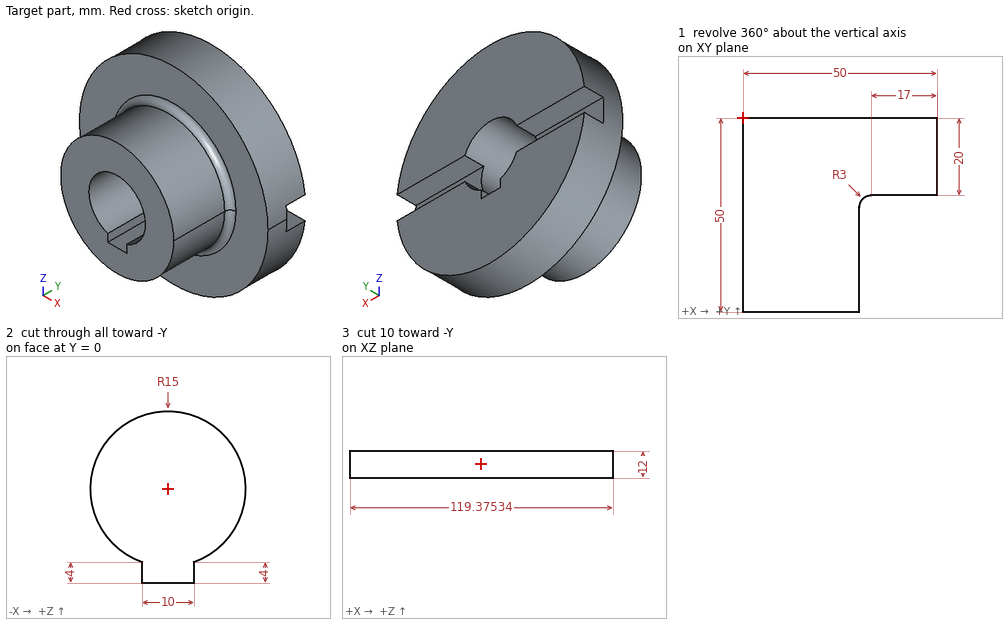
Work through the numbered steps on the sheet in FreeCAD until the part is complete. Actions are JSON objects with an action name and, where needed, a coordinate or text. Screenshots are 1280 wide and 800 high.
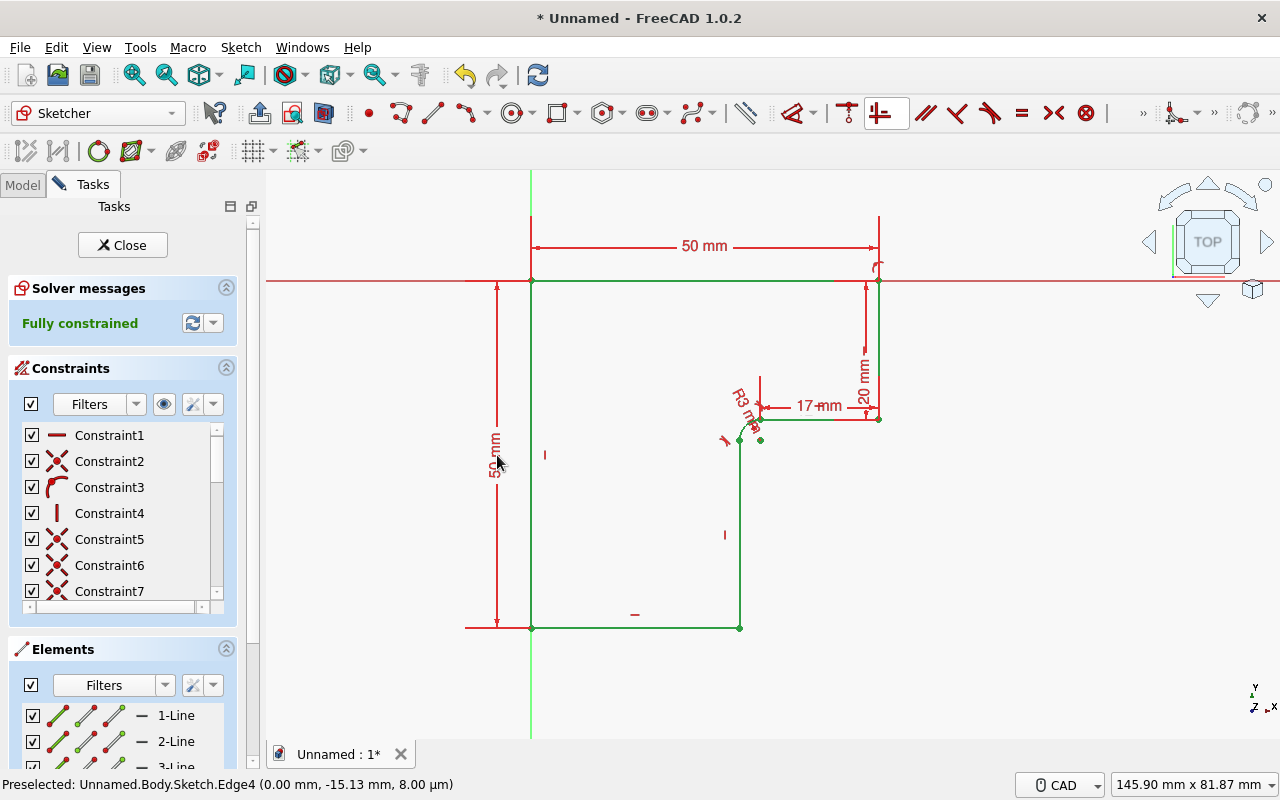
{"action": "left_click", "coordinate": [123, 245]}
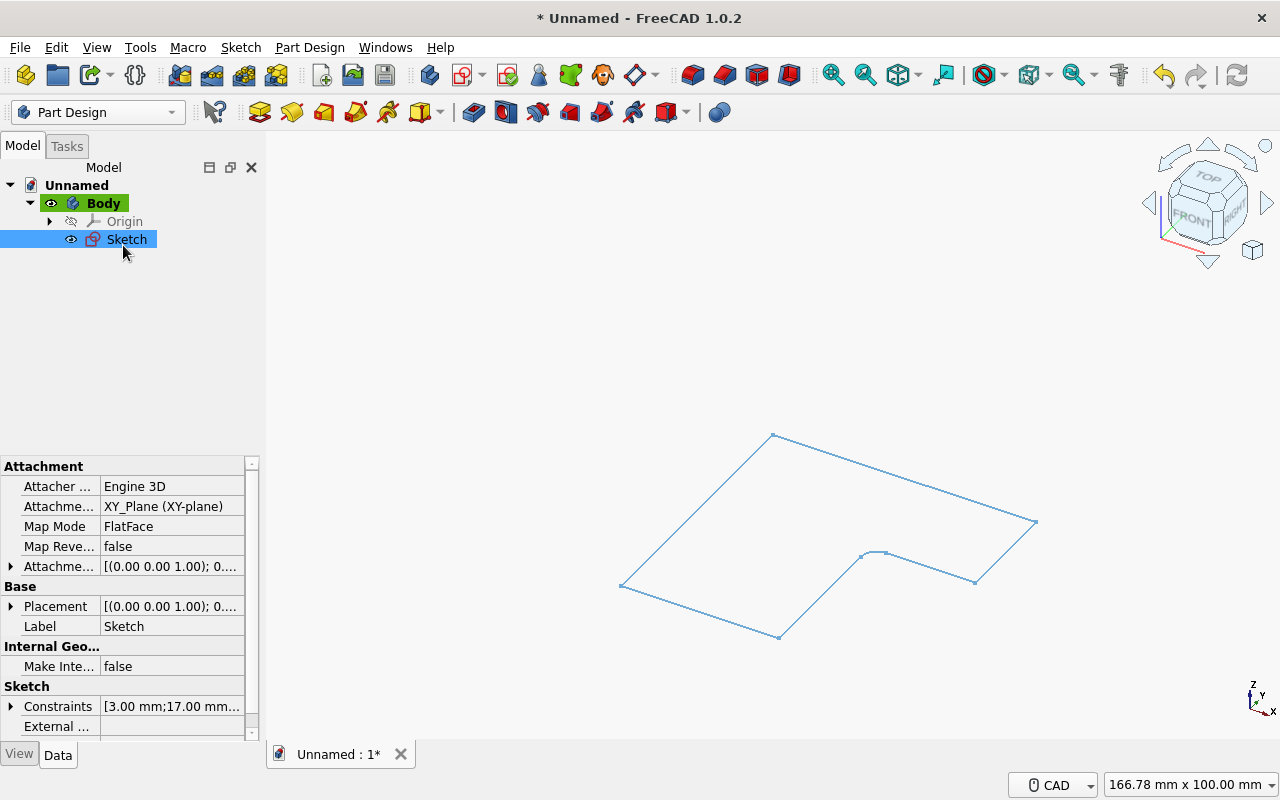
{"action": "left_click", "coordinate": [292, 112]}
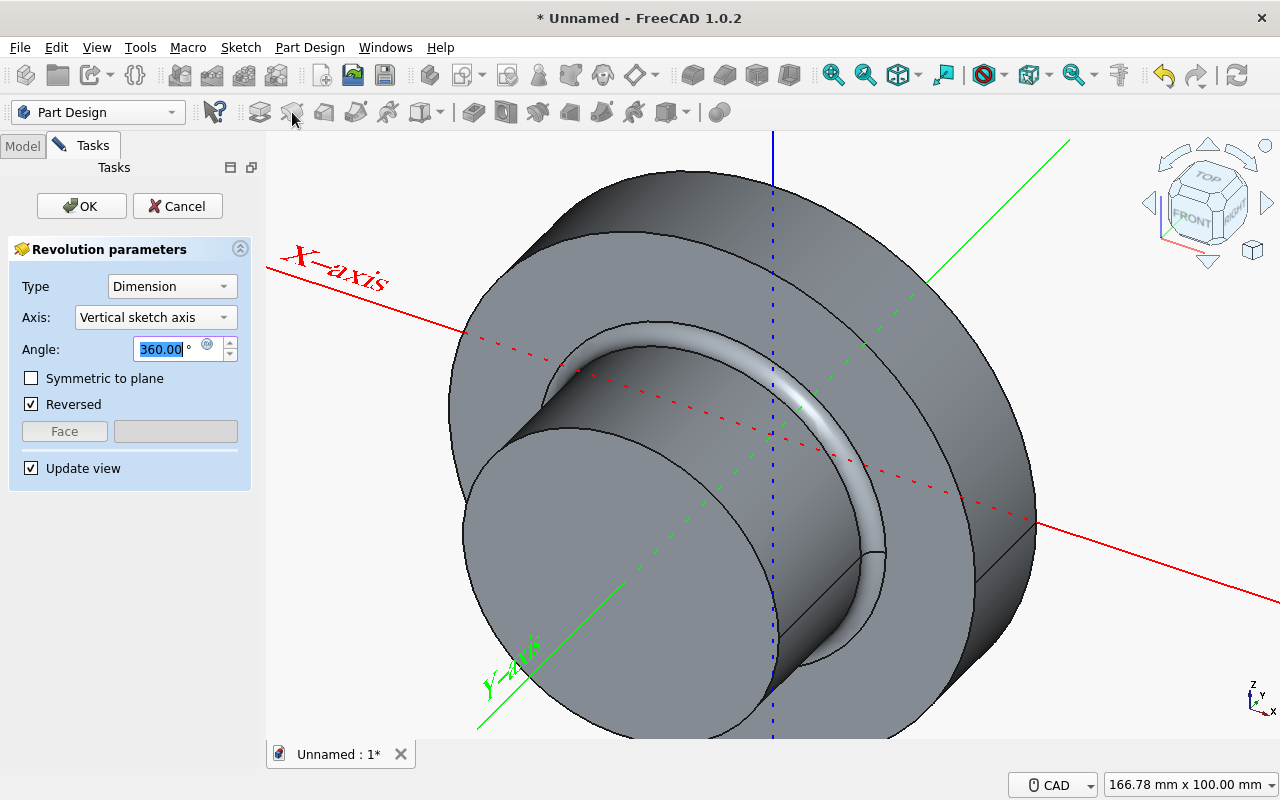
{"action": "left_click", "coordinate": [82, 206]}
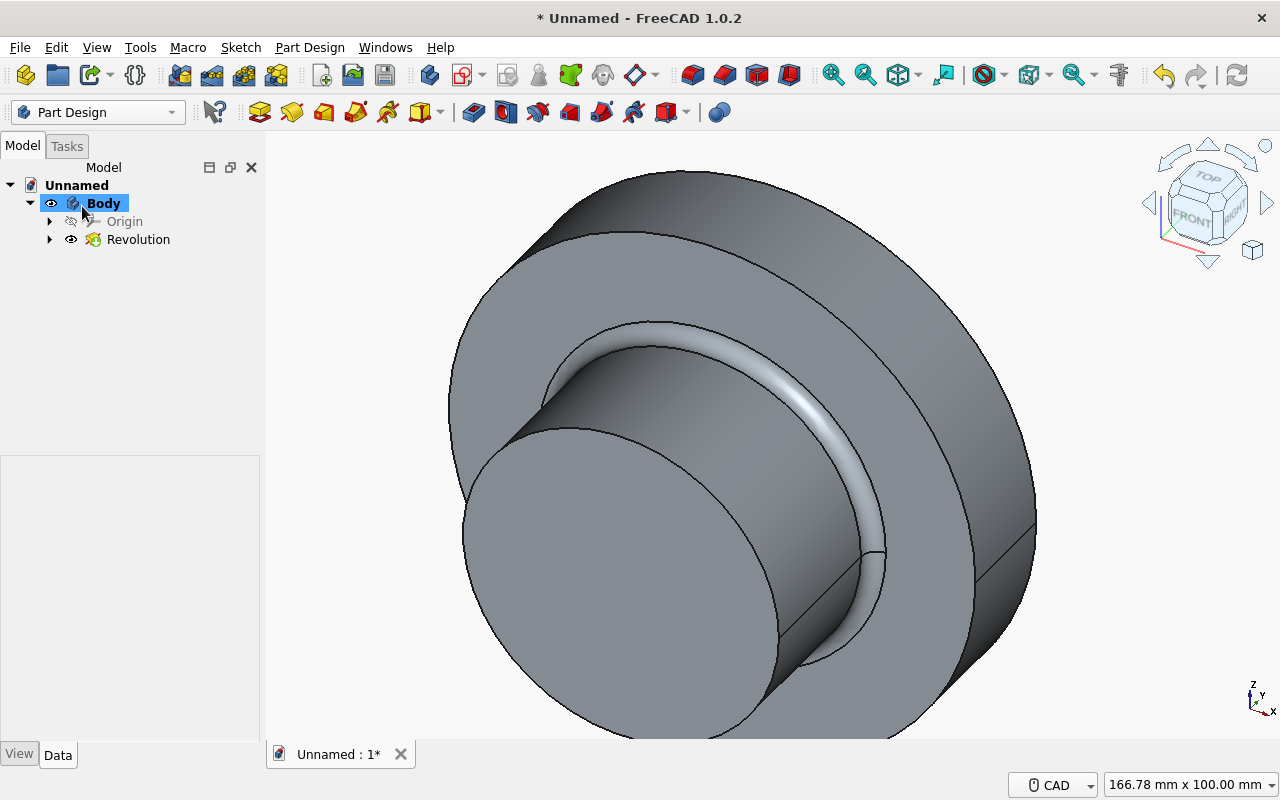
{"action": "left_click", "coordinate": [834, 76]}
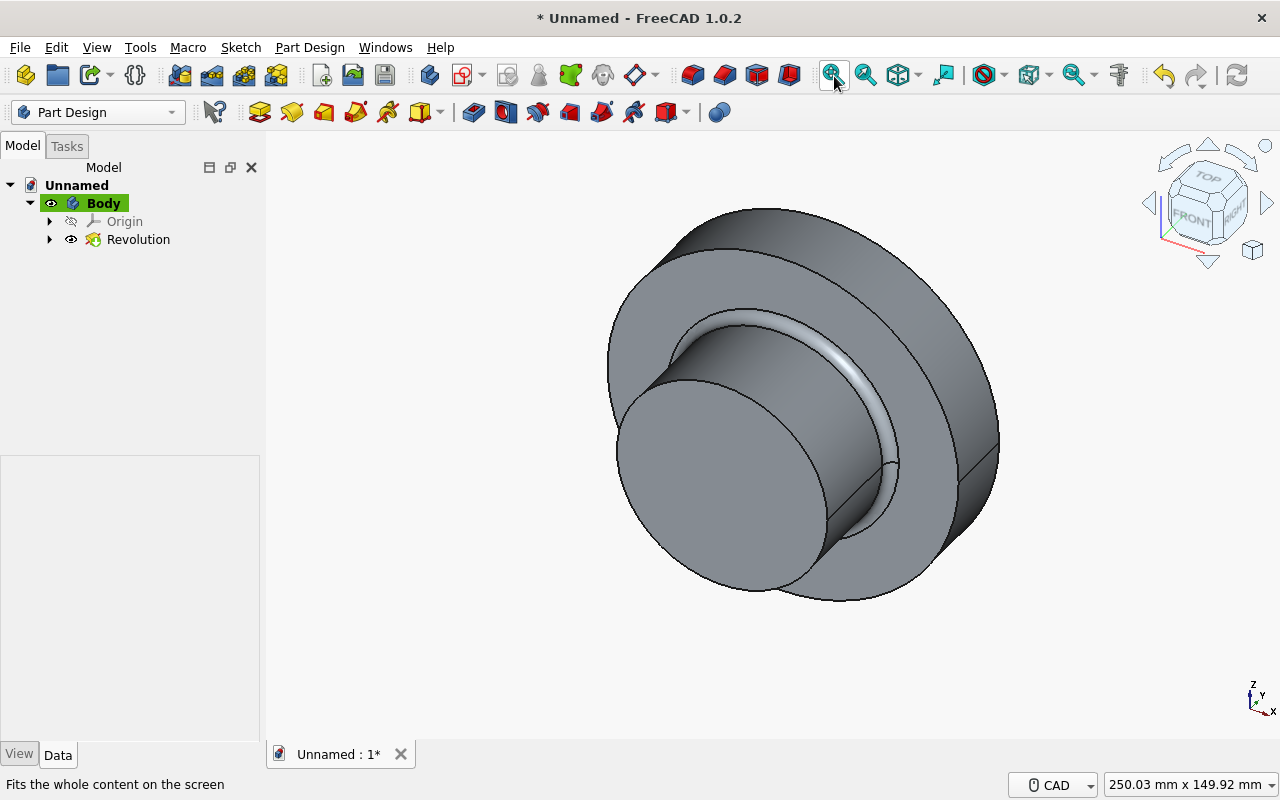
{"action": "key", "text": "4"}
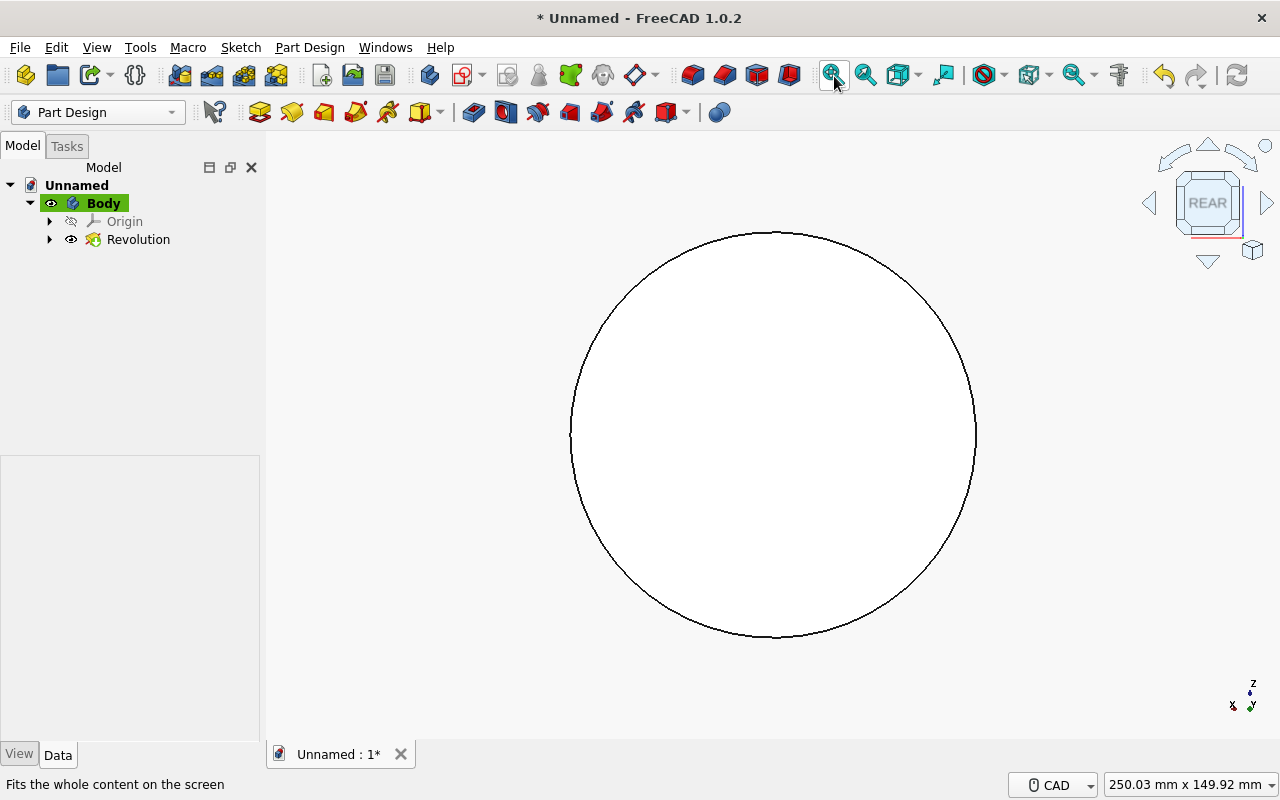
{"action": "left_click", "coordinate": [773, 434]}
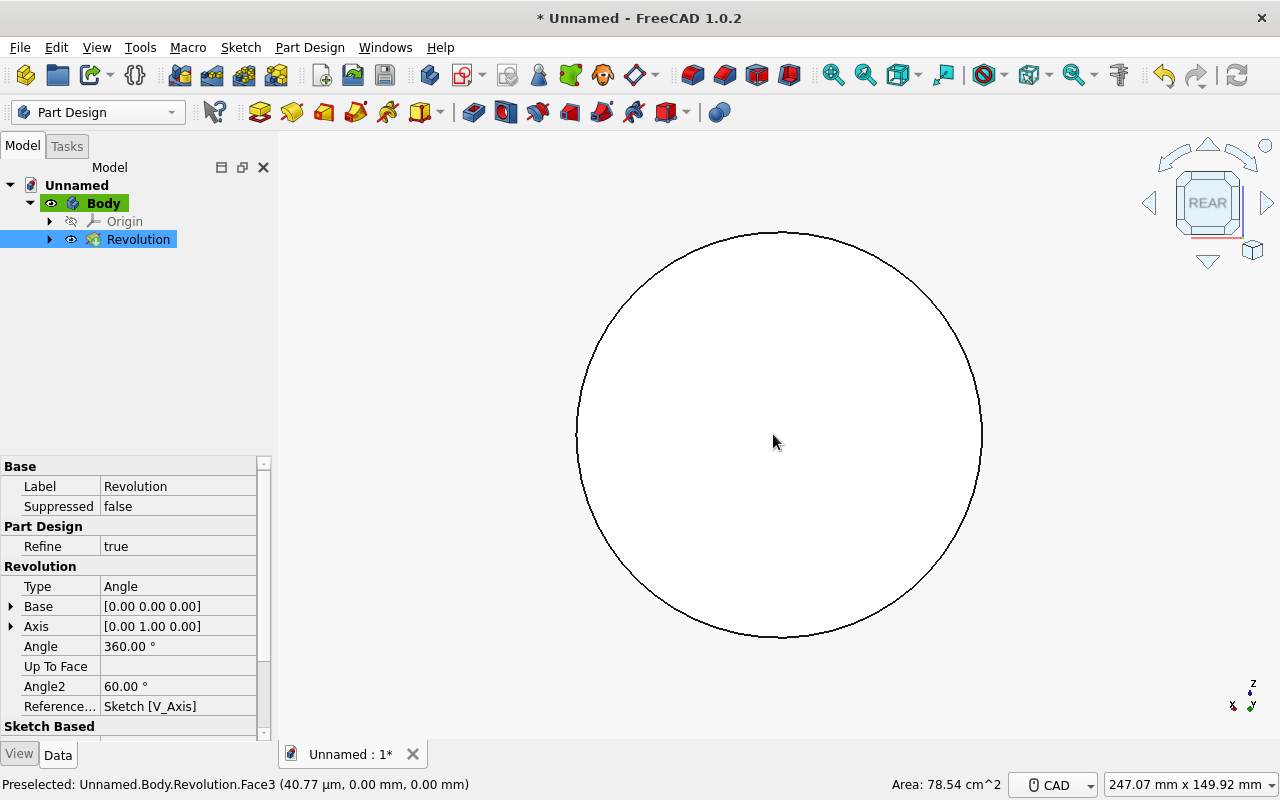
{"action": "left_click", "coordinate": [462, 76]}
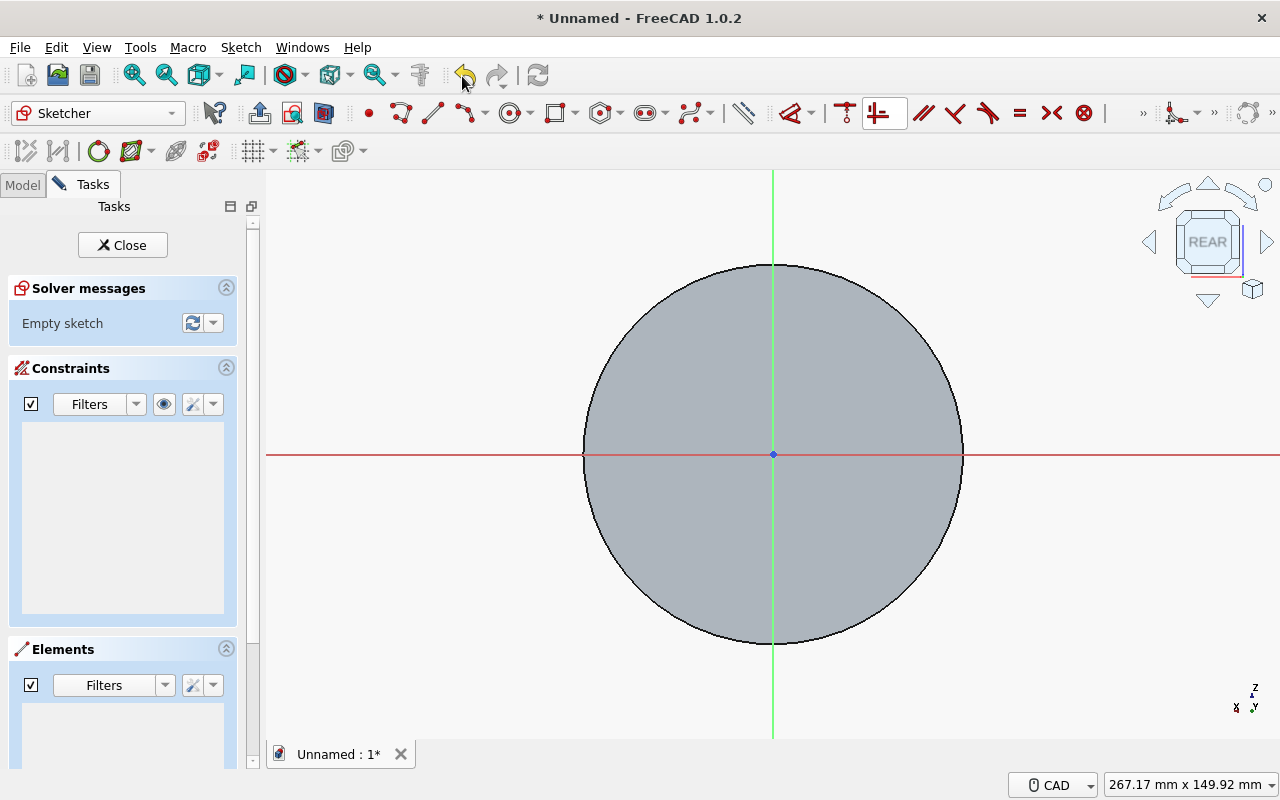
{"action": "scroll", "coordinate": [813, 464], "scroll_direction": "up", "scroll_amount": 5}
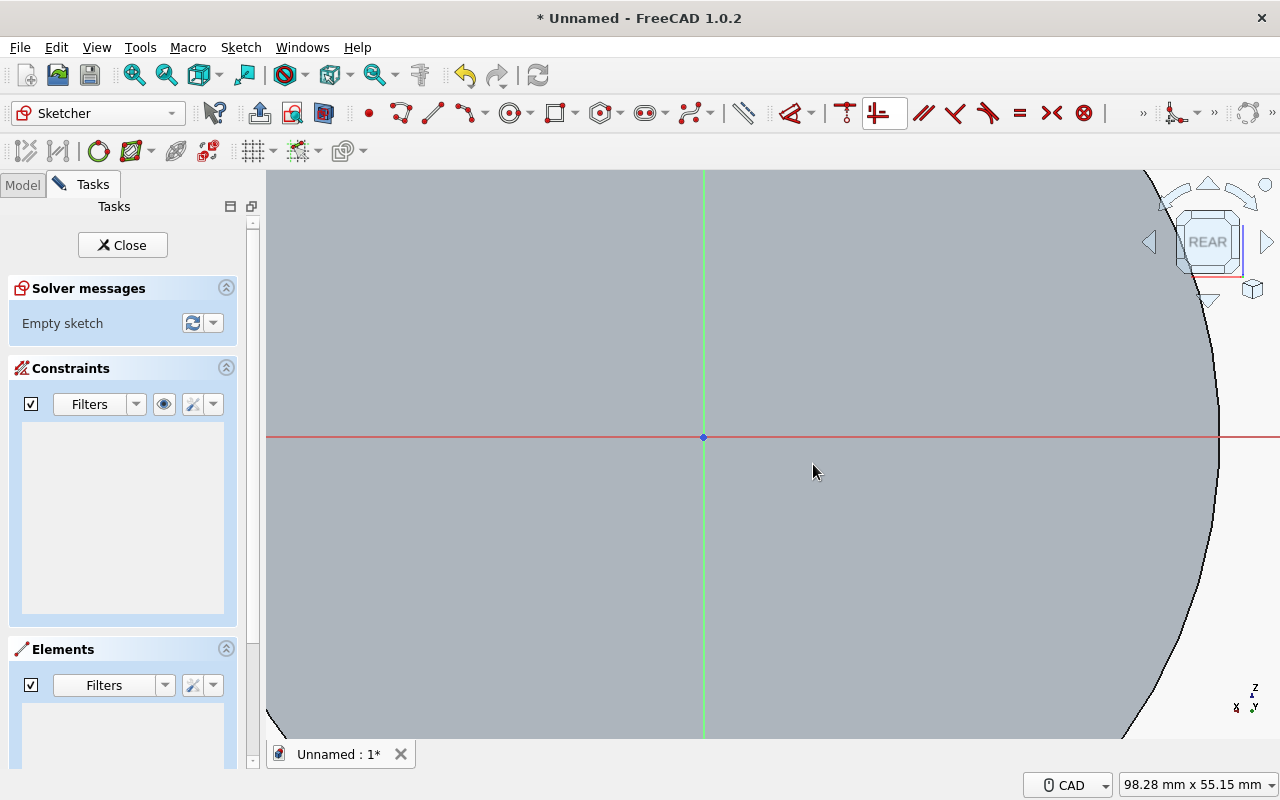
{"action": "left_click", "coordinate": [402, 114]}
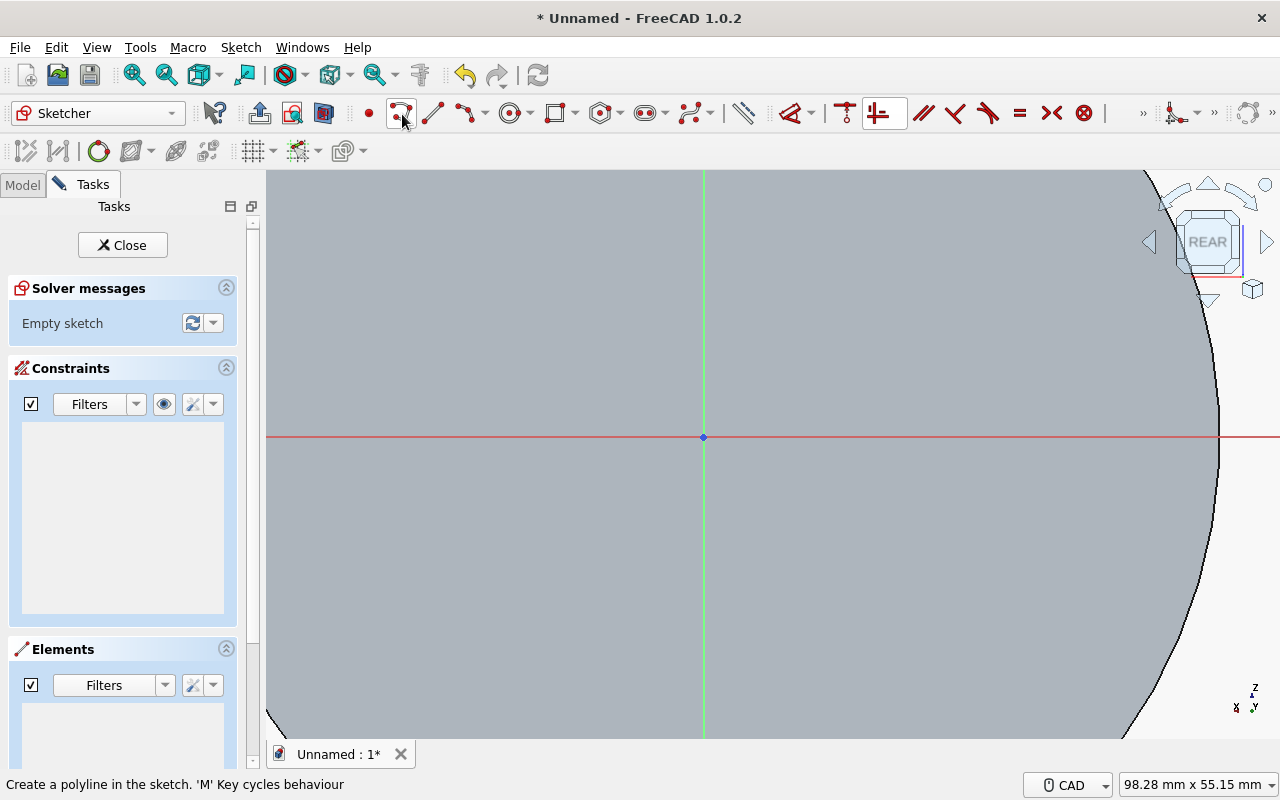
{"action": "left_click", "coordinate": [652, 583]}
{"action": "left_click", "coordinate": [652, 624]}
{"action": "left_click", "coordinate": [755, 624]}
{"action": "left_click", "coordinate": [755, 583]}
{"action": "right_click", "coordinate": [755, 583]}